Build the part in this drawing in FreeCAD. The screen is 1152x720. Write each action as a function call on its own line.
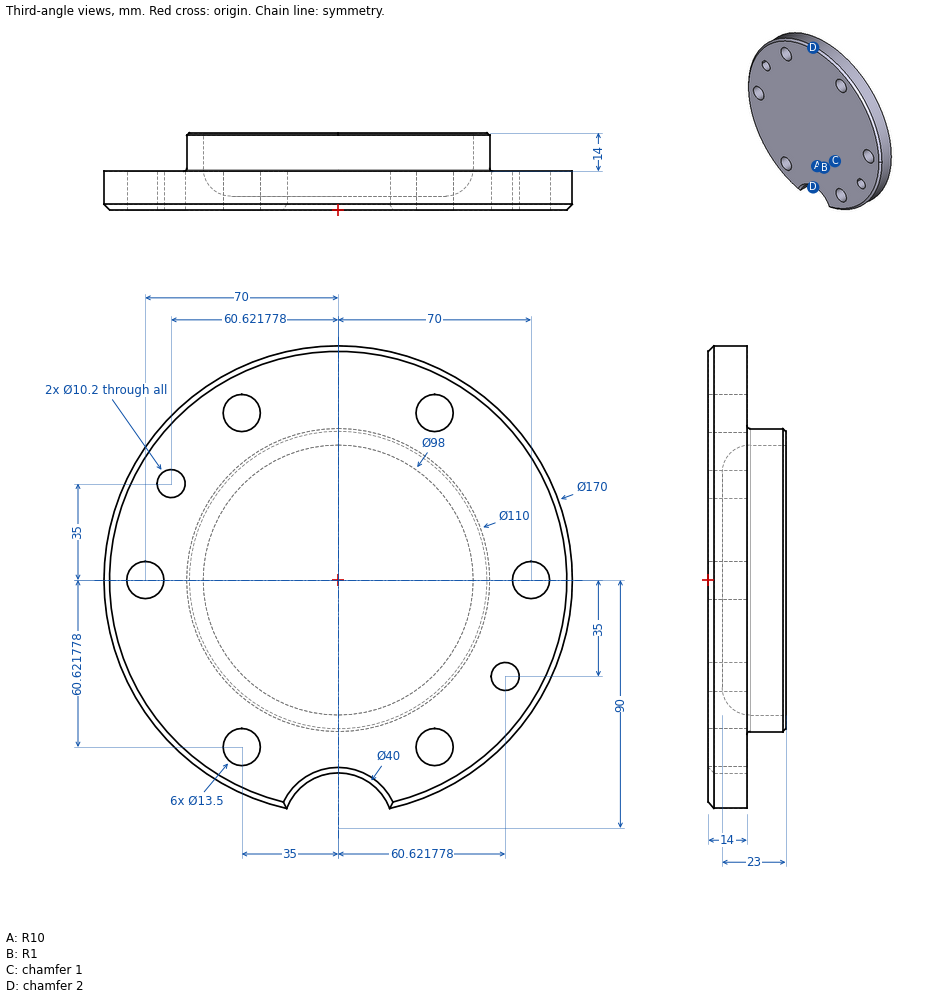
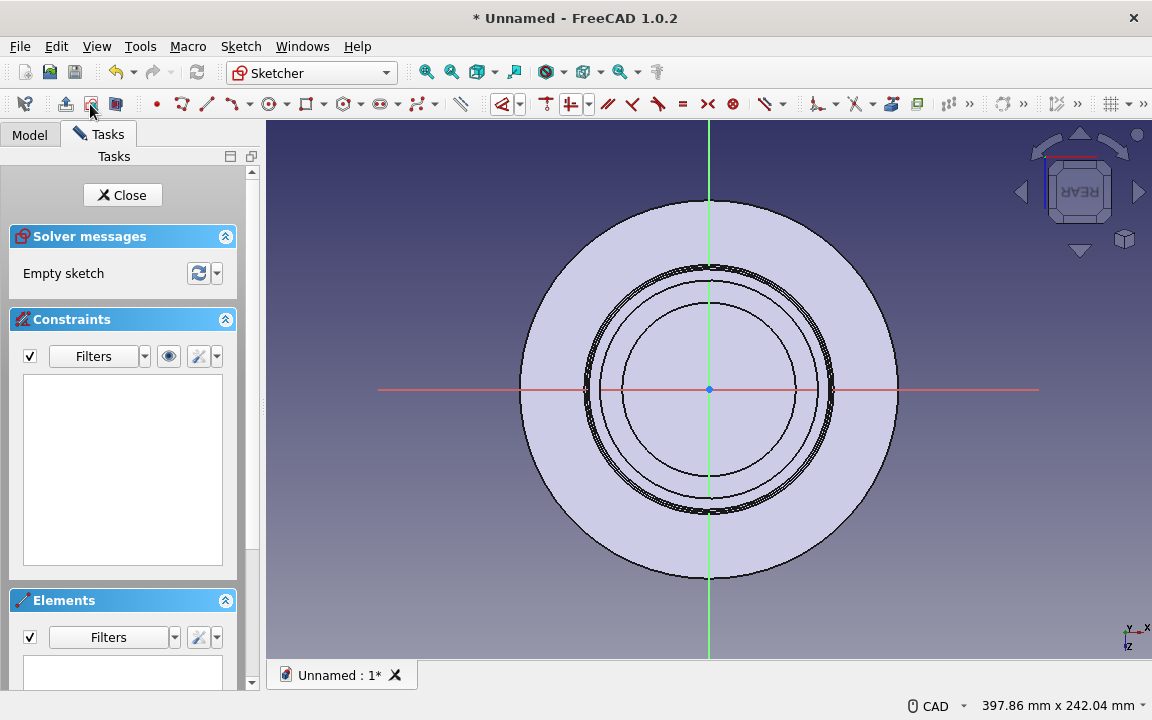
scroll(331, 604, down, 1)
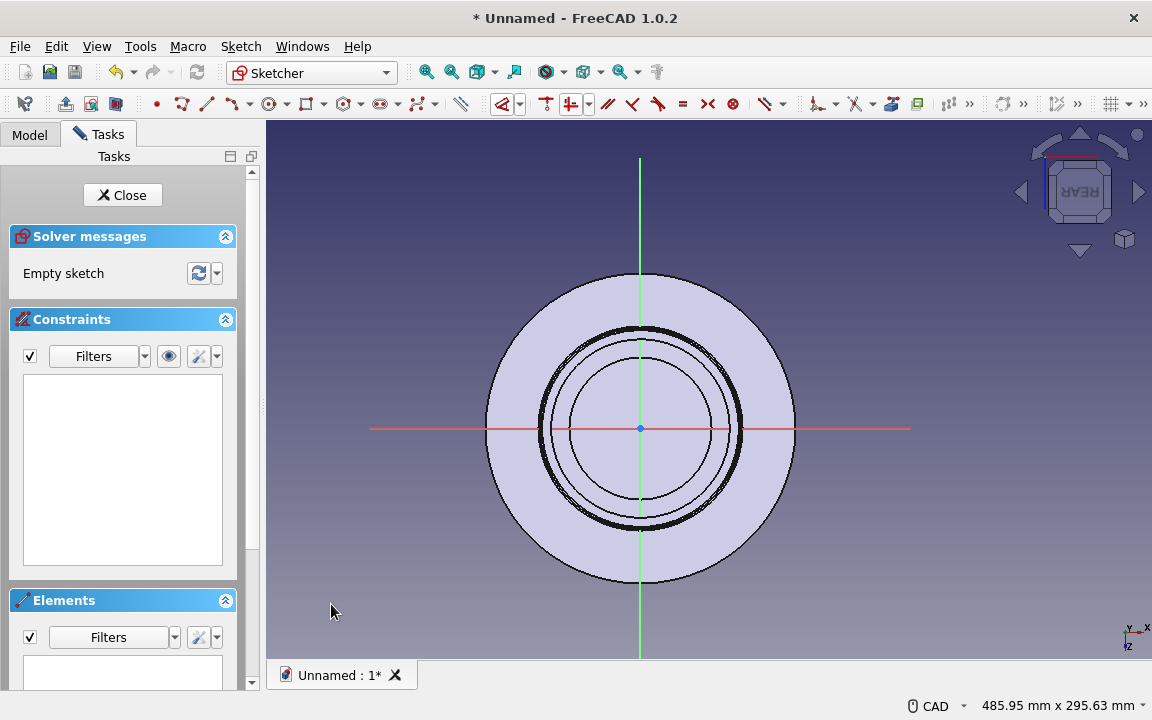
click(268, 104)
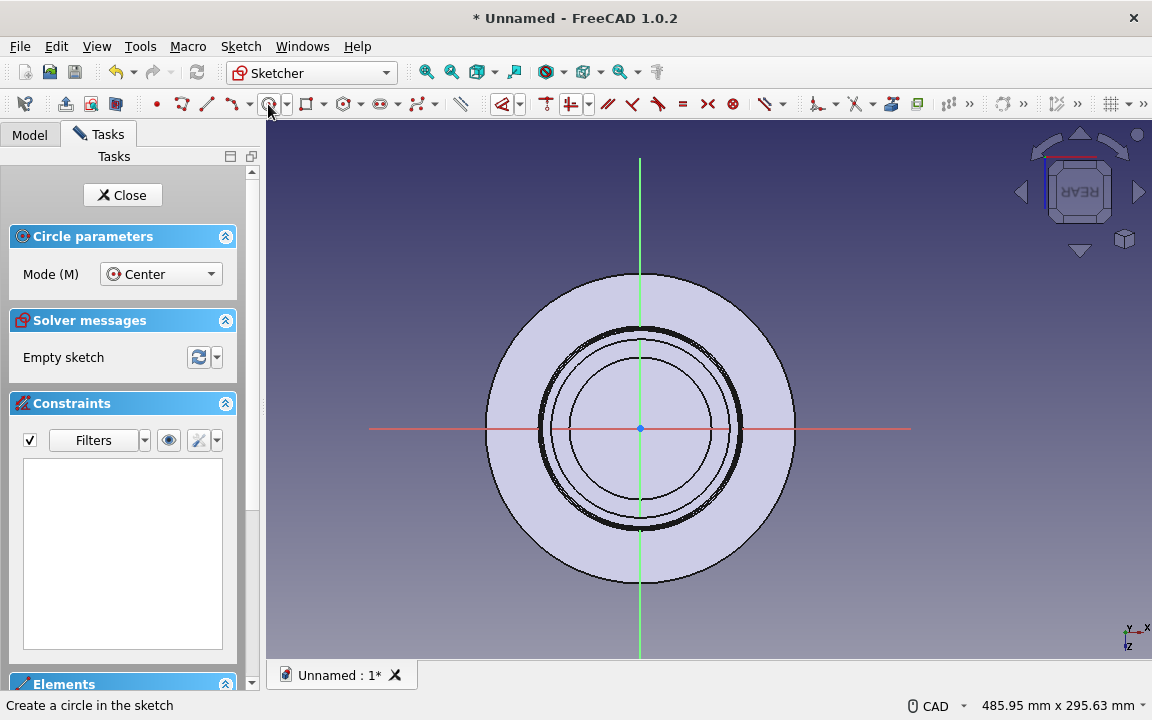
click(640, 264)
click(666, 239)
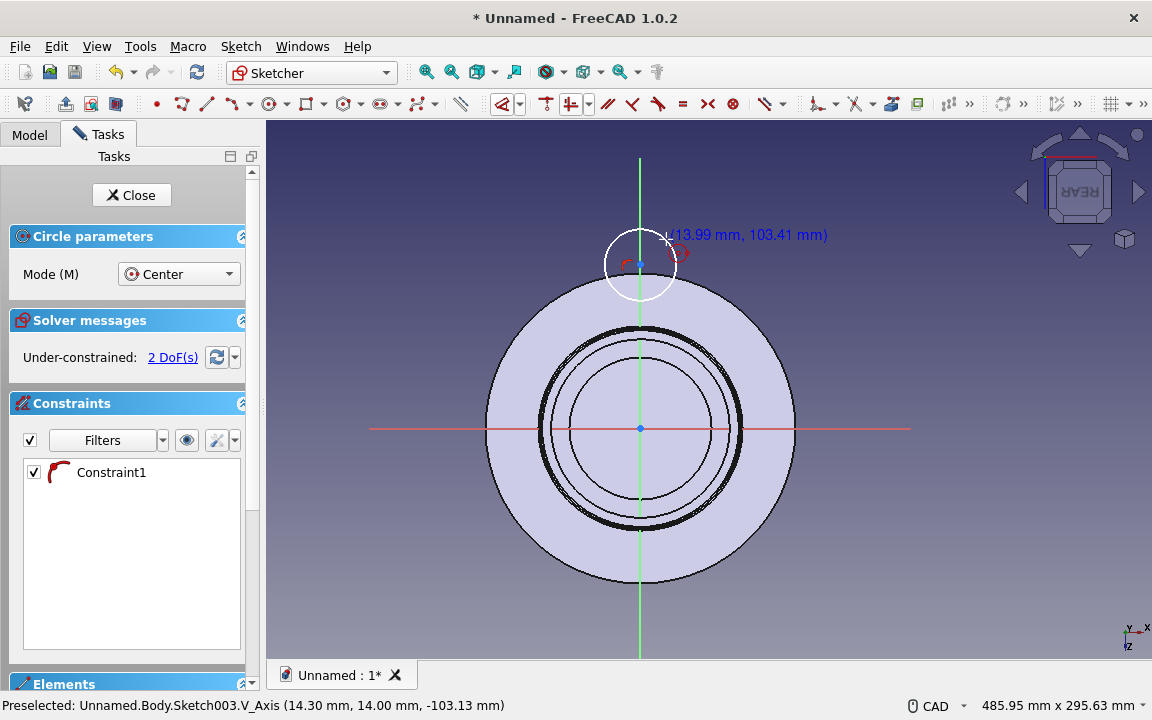
scroll(577, 318, up, 4)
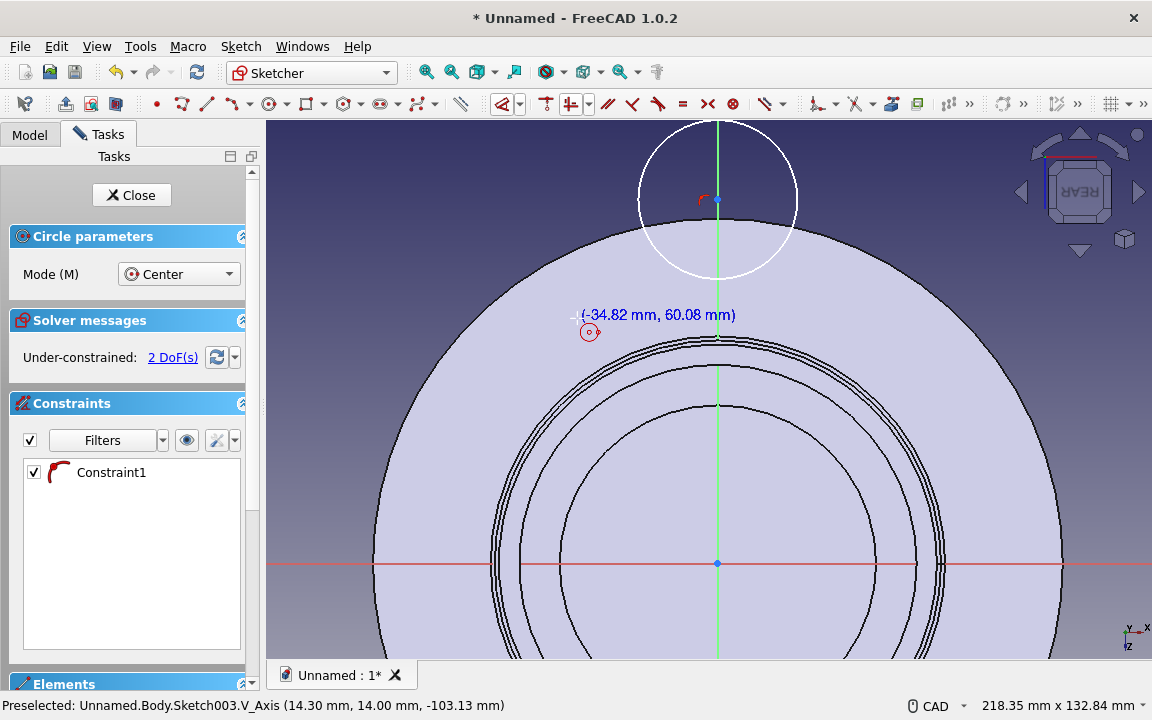
click(576, 318)
click(595, 298)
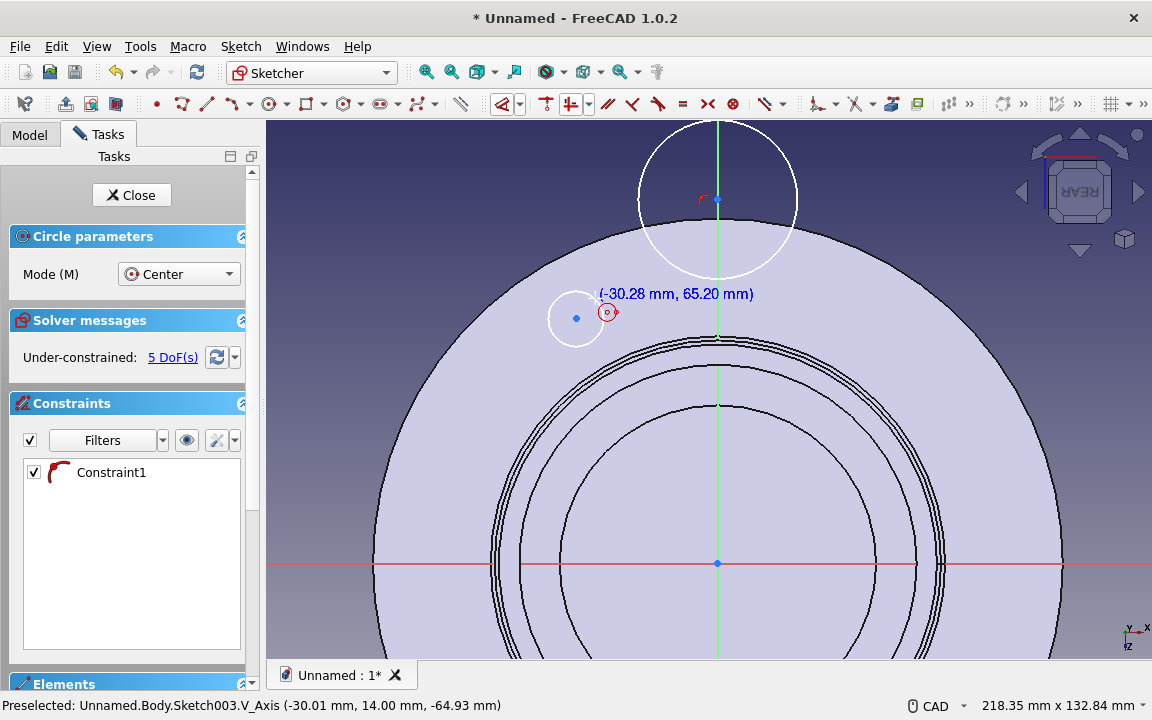
click(860, 318)
click(879, 298)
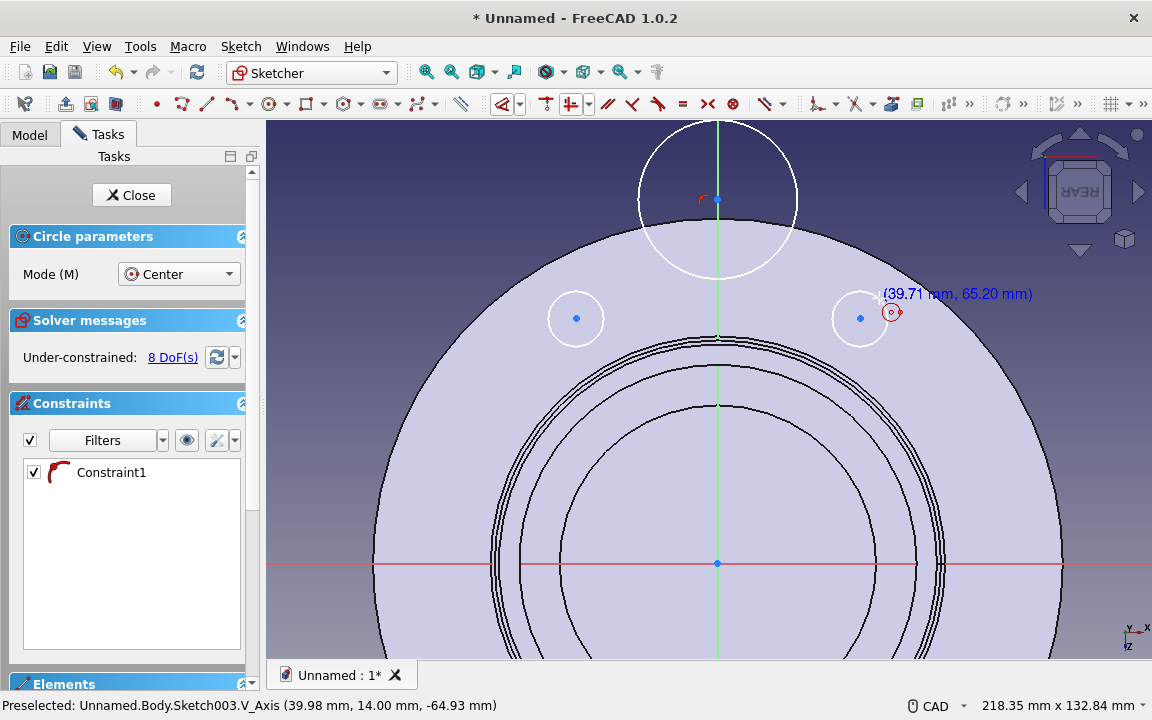
scroll(577, 318, down, 4)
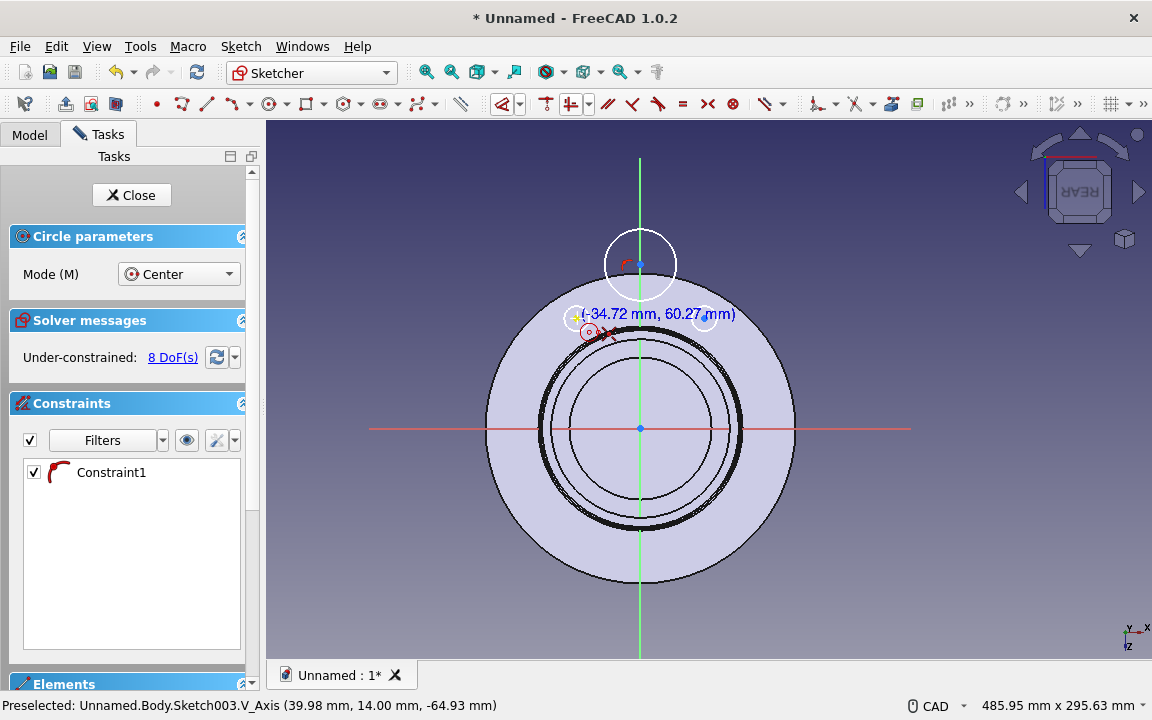
scroll(768, 429, up, 4)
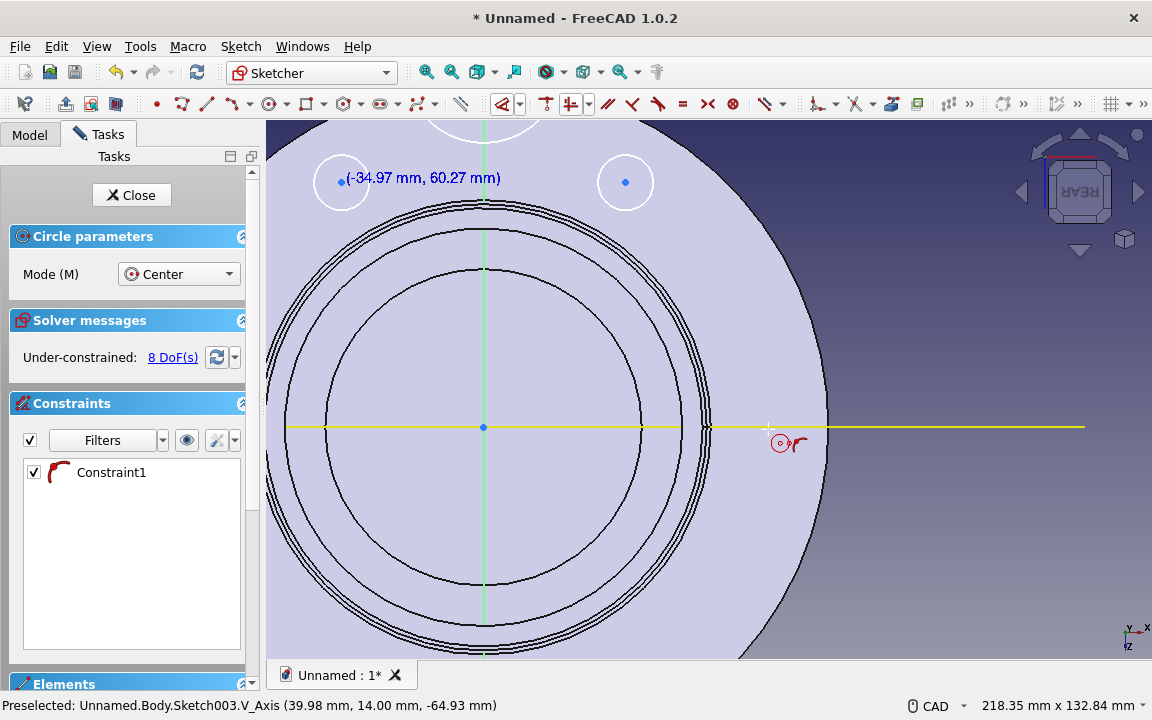
click(768, 427)
click(787, 408)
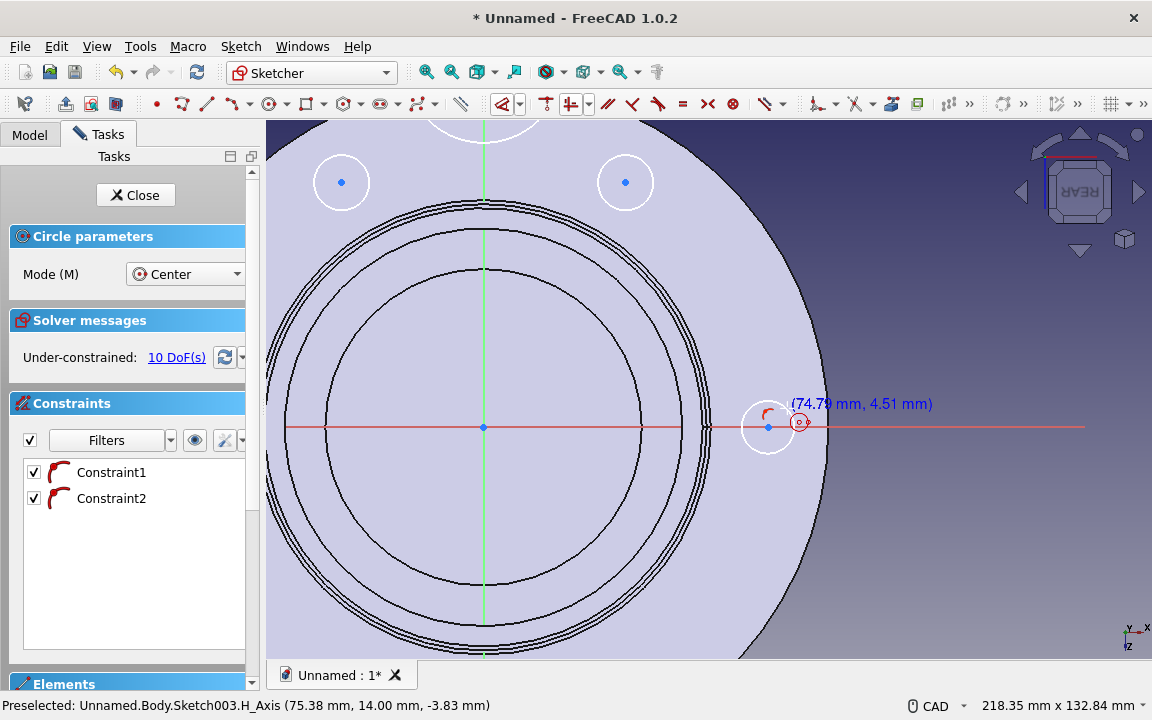
scroll(769, 429, down, 4)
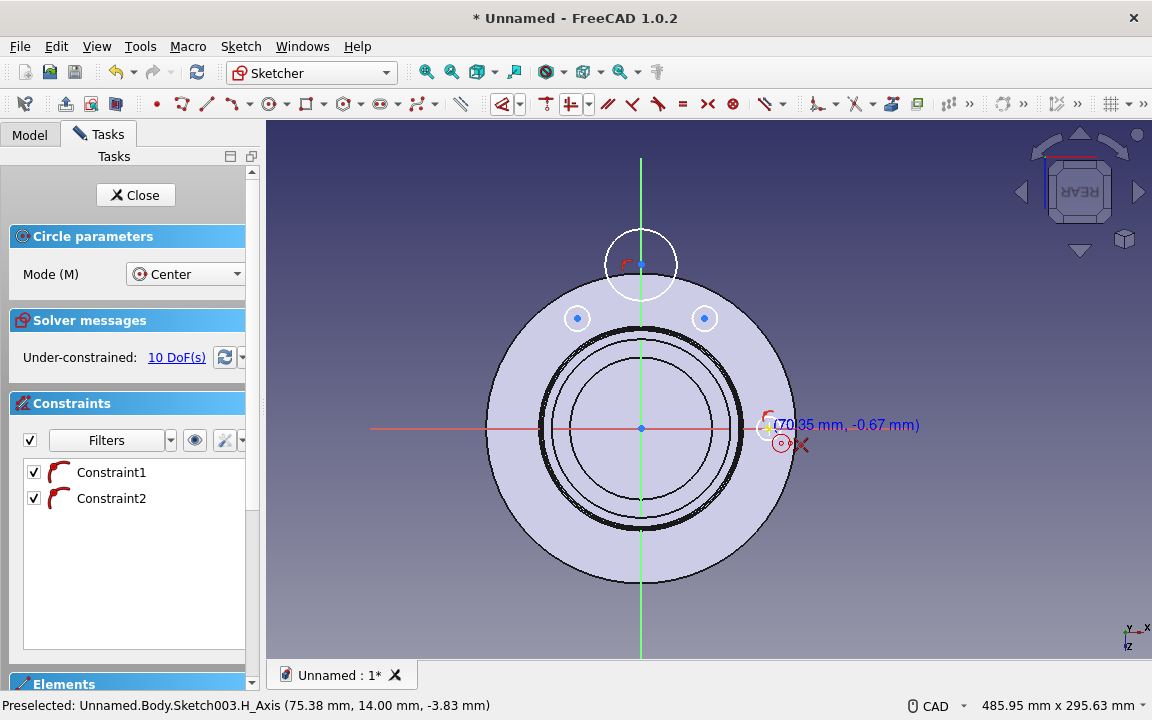
scroll(705, 539, up, 4)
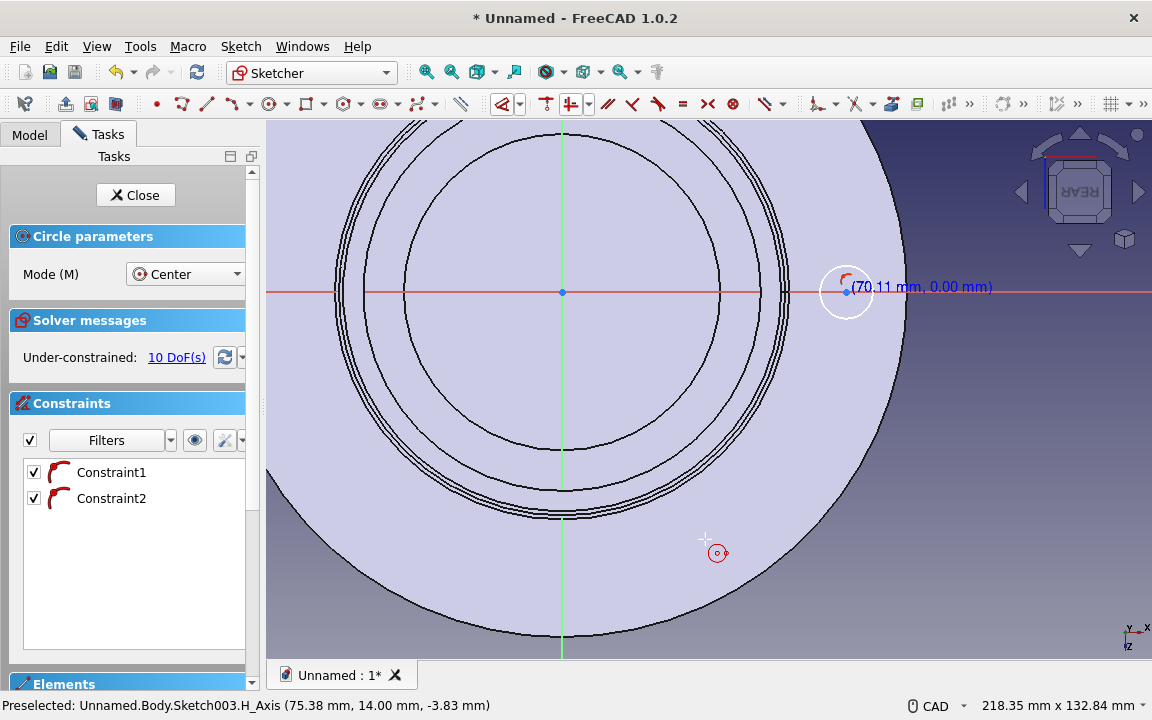
click(704, 538)
click(723, 519)